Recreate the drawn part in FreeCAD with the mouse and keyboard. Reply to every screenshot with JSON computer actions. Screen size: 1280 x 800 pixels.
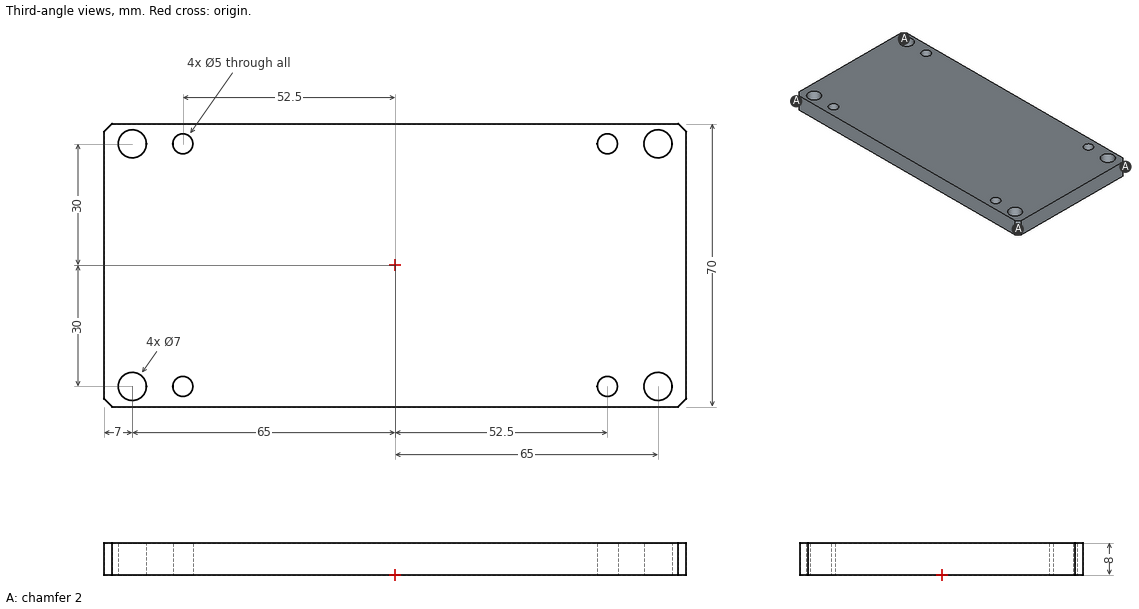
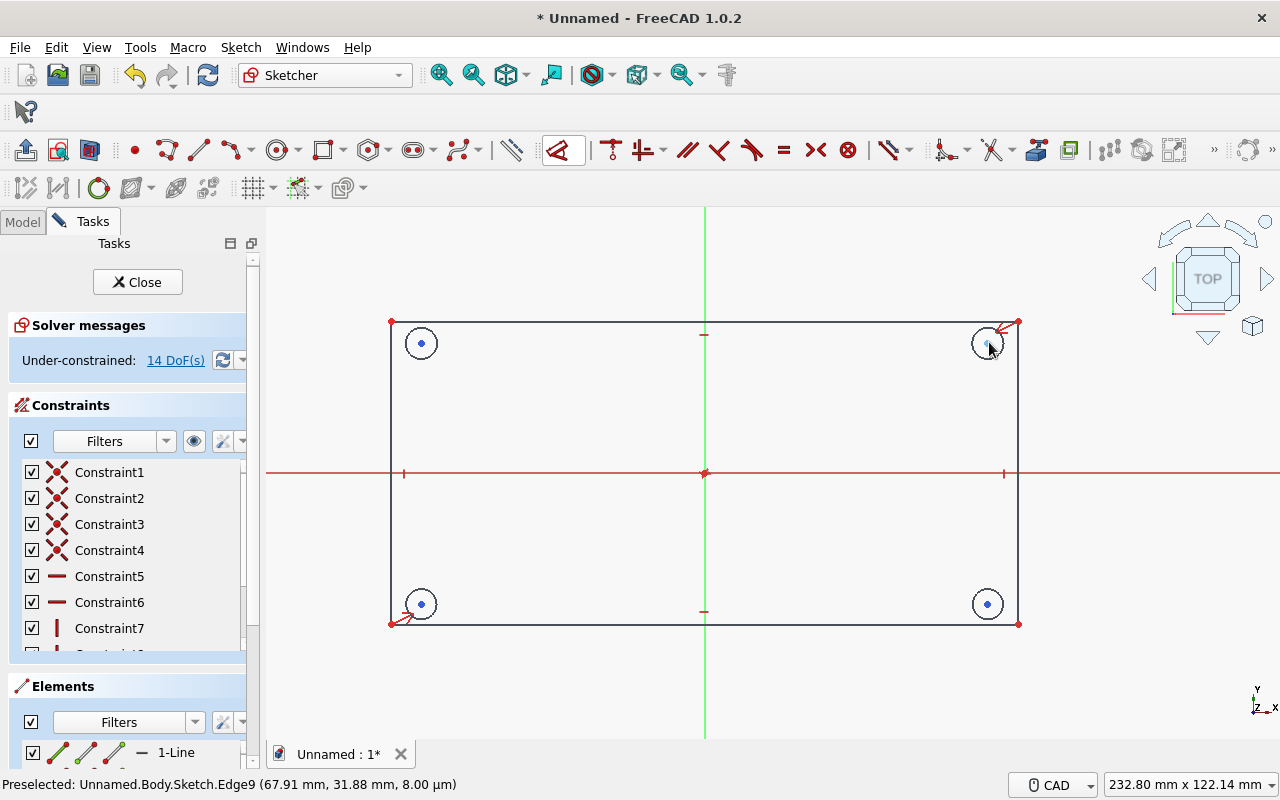
{"action": "left_click", "coordinate": [432, 593]}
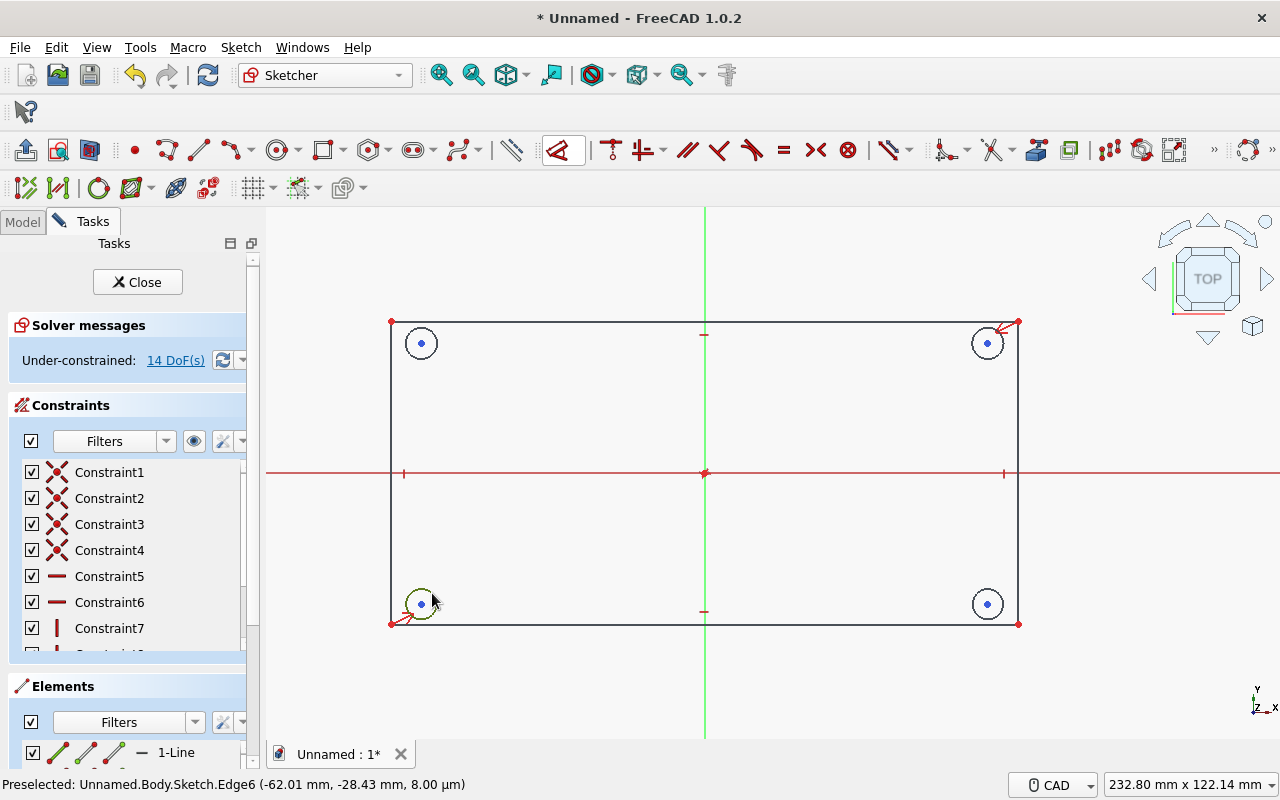
{"action": "left_click", "coordinate": [999, 593]}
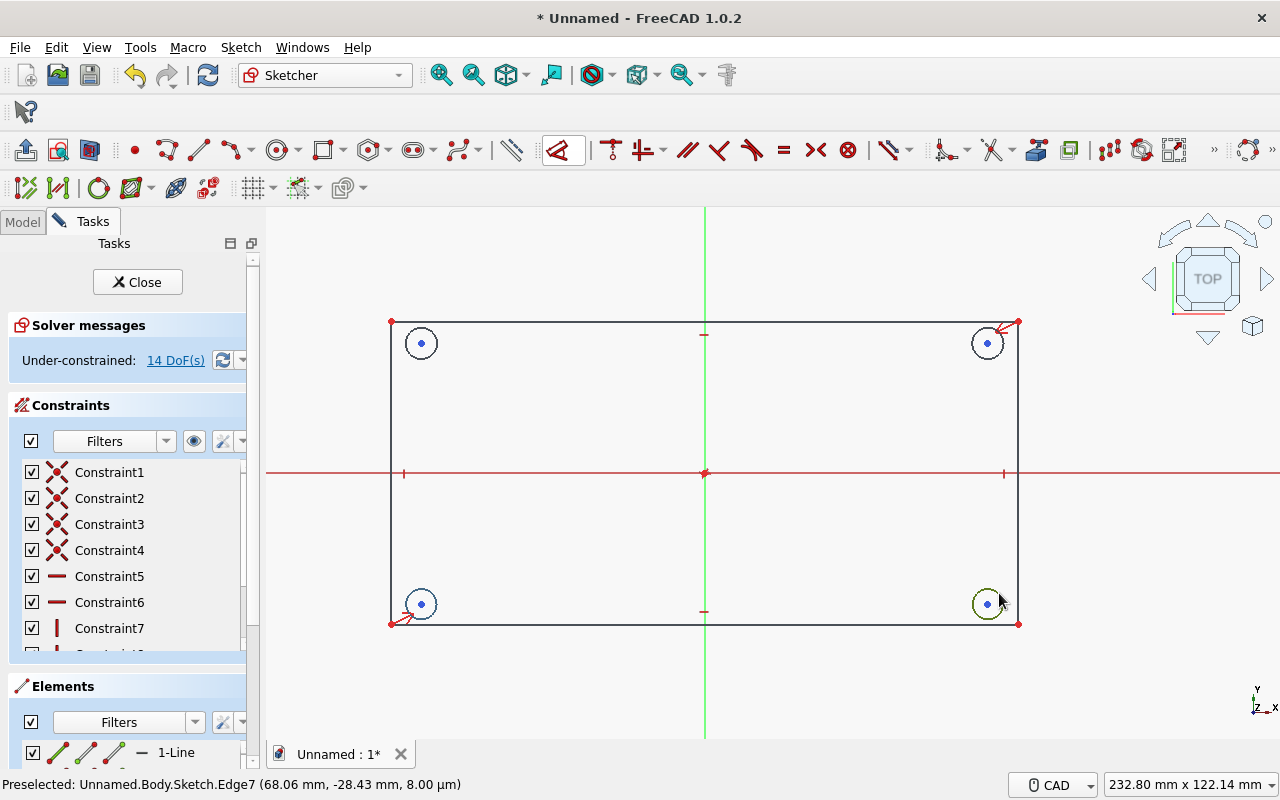
{"action": "scroll", "coordinate": [432, 332], "scroll_direction": "up", "scroll_amount": 2}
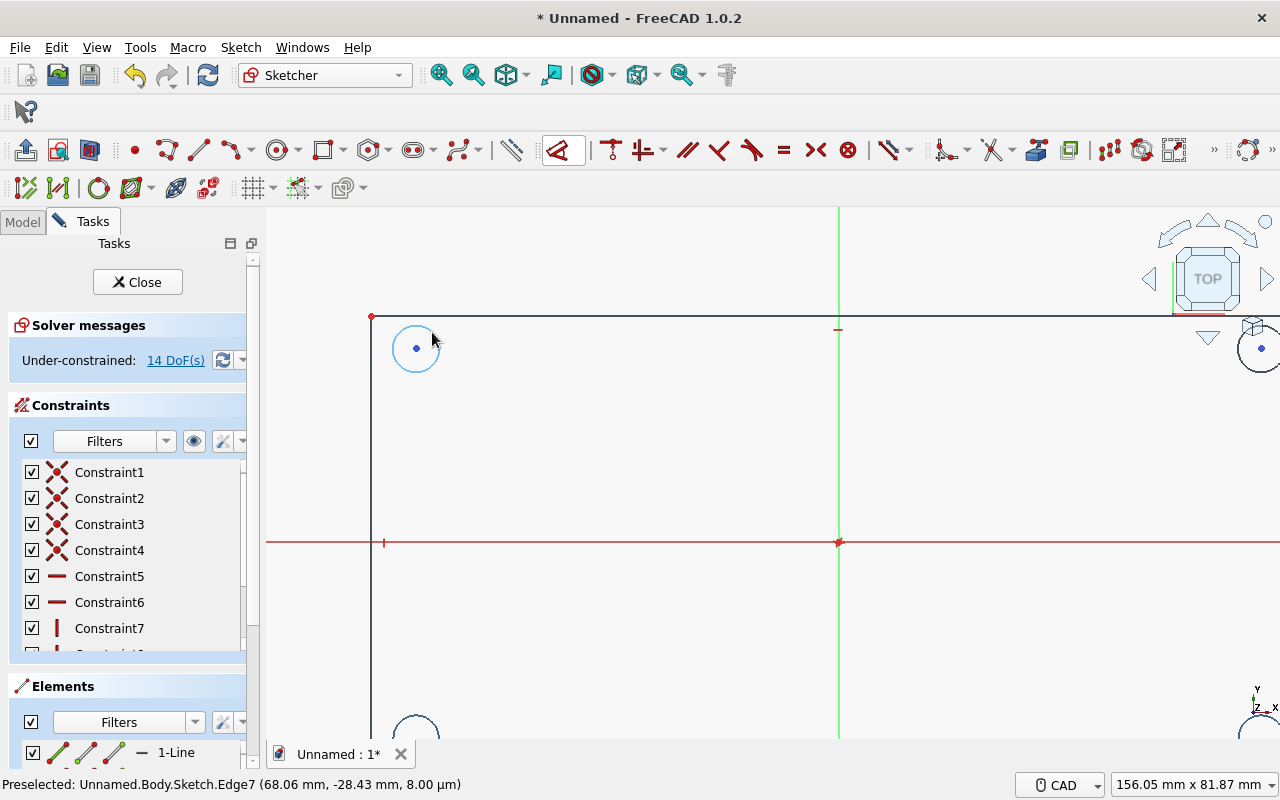
{"action": "left_click", "coordinate": [433, 332]}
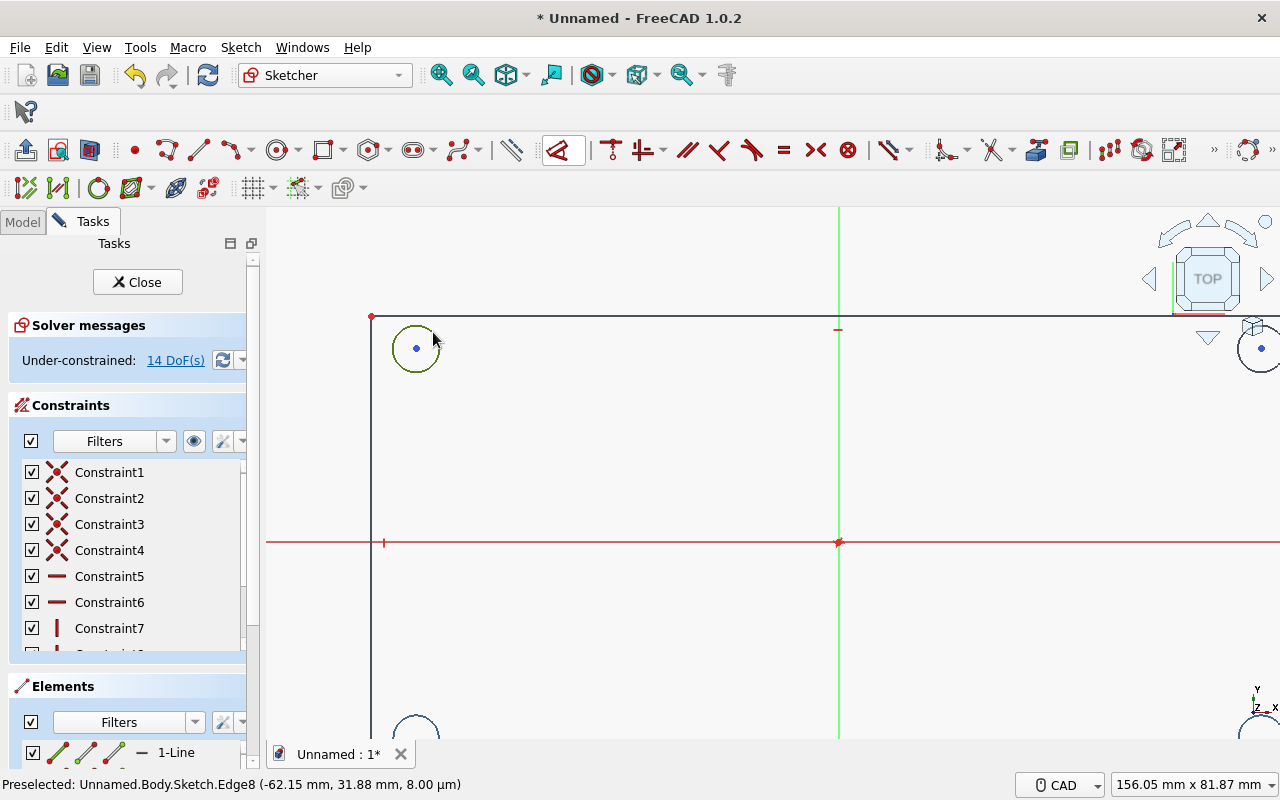
{"action": "scroll", "coordinate": [431, 332], "scroll_direction": "down", "scroll_amount": 2}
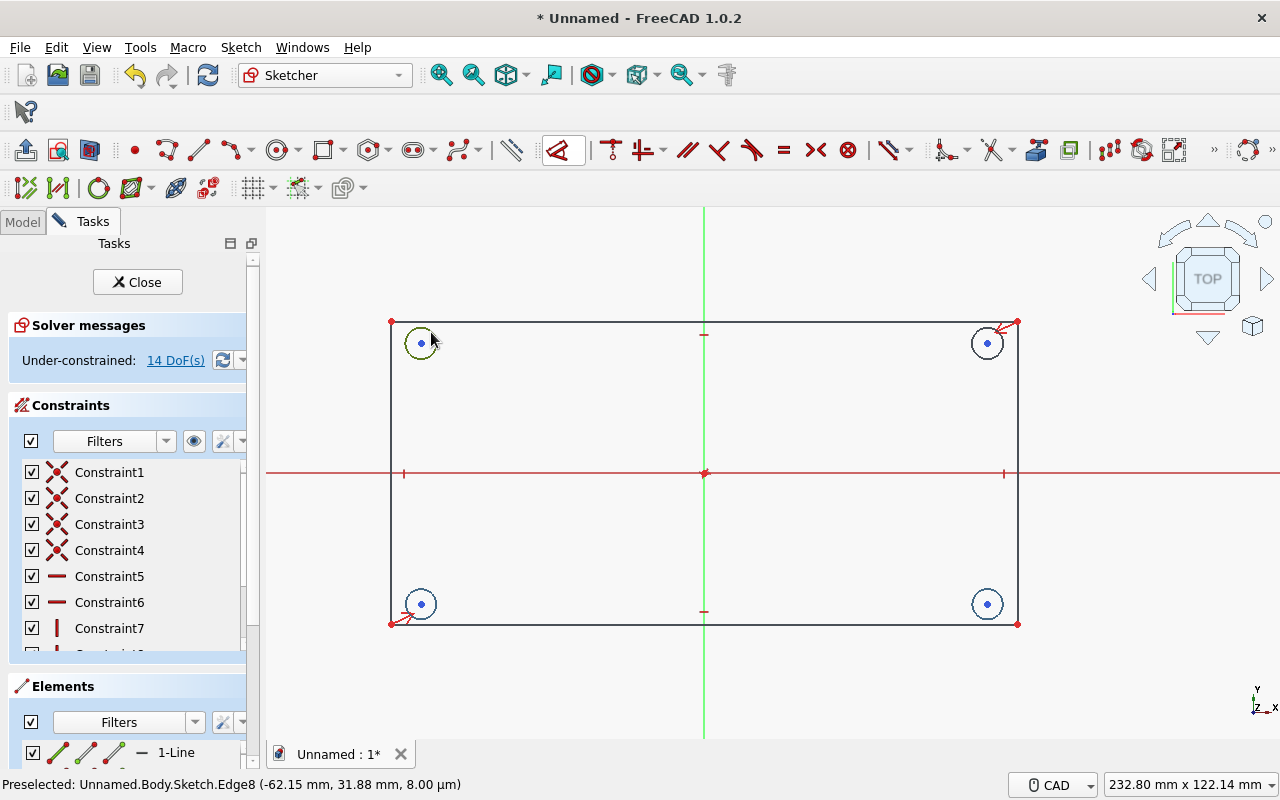
{"action": "scroll", "coordinate": [999, 332], "scroll_direction": "up", "scroll_amount": 2}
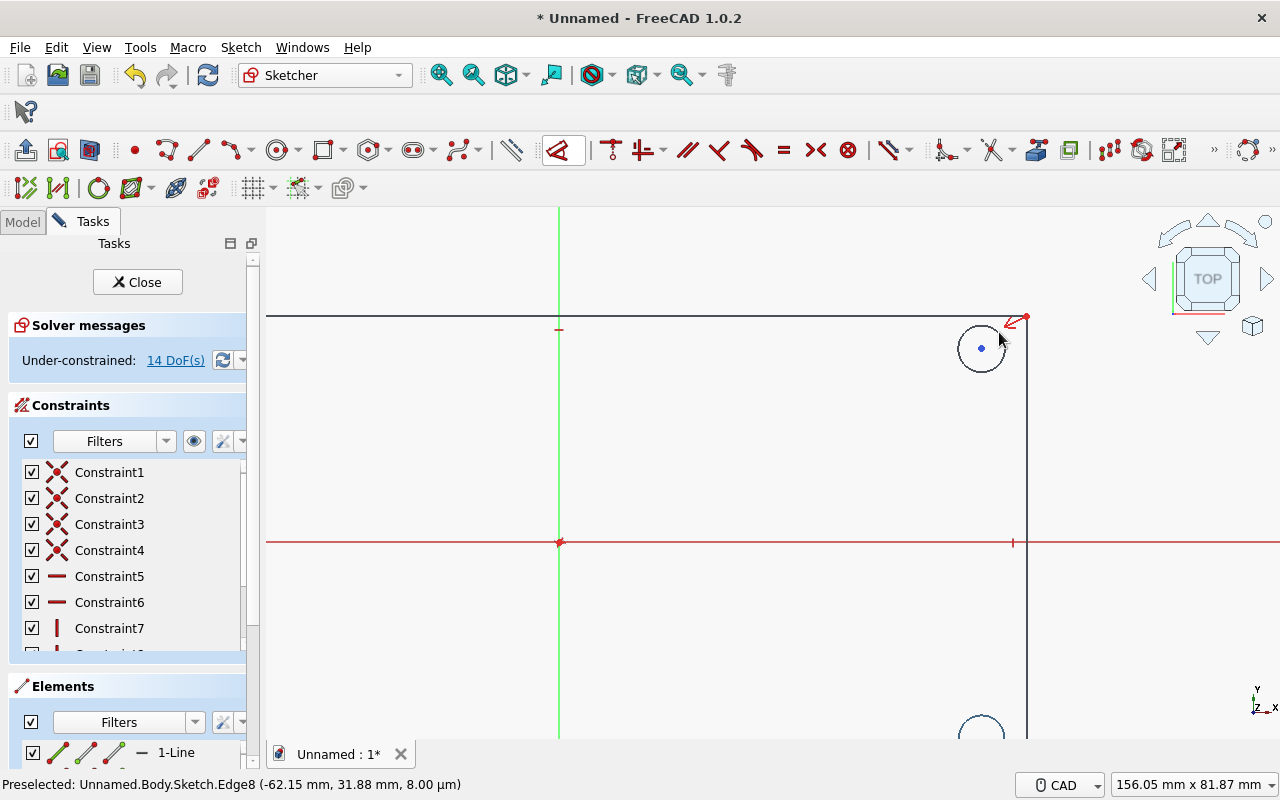
{"action": "left_click", "coordinate": [998, 332]}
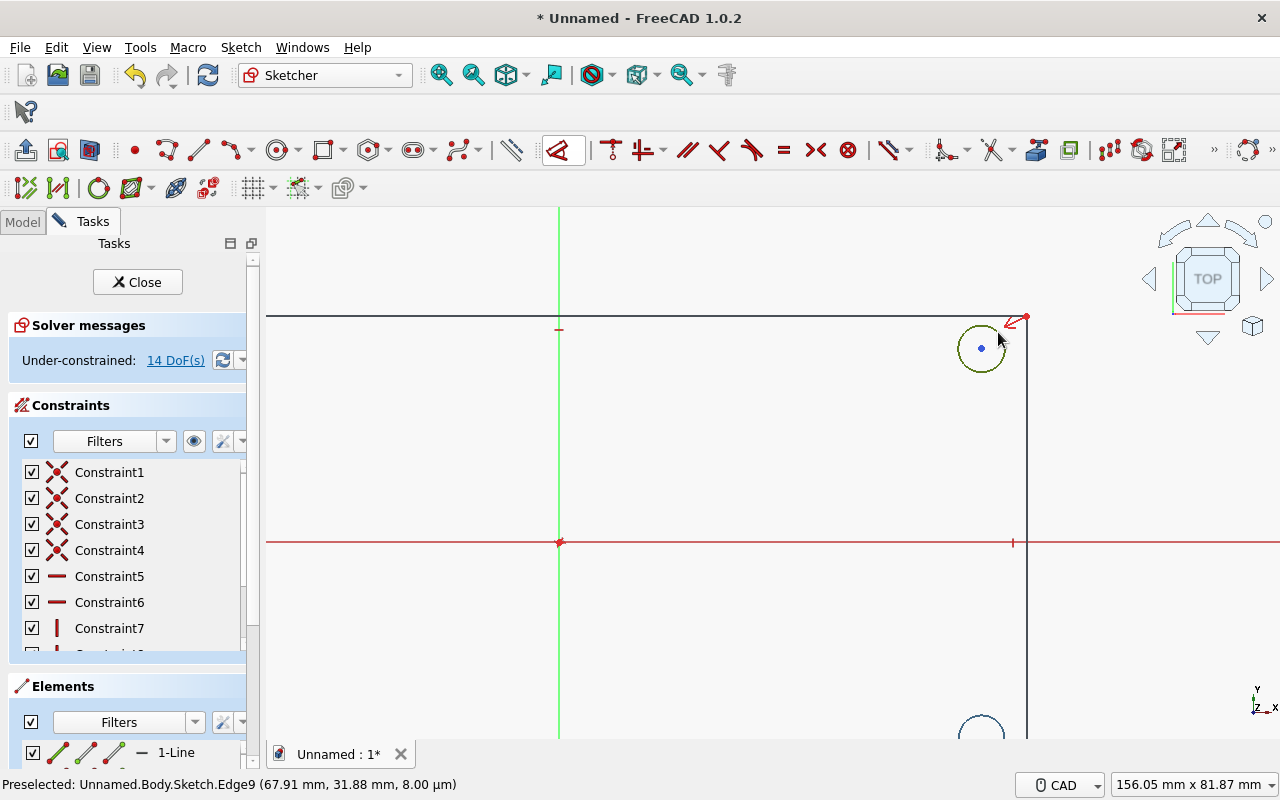
{"action": "left_click", "coordinate": [784, 150]}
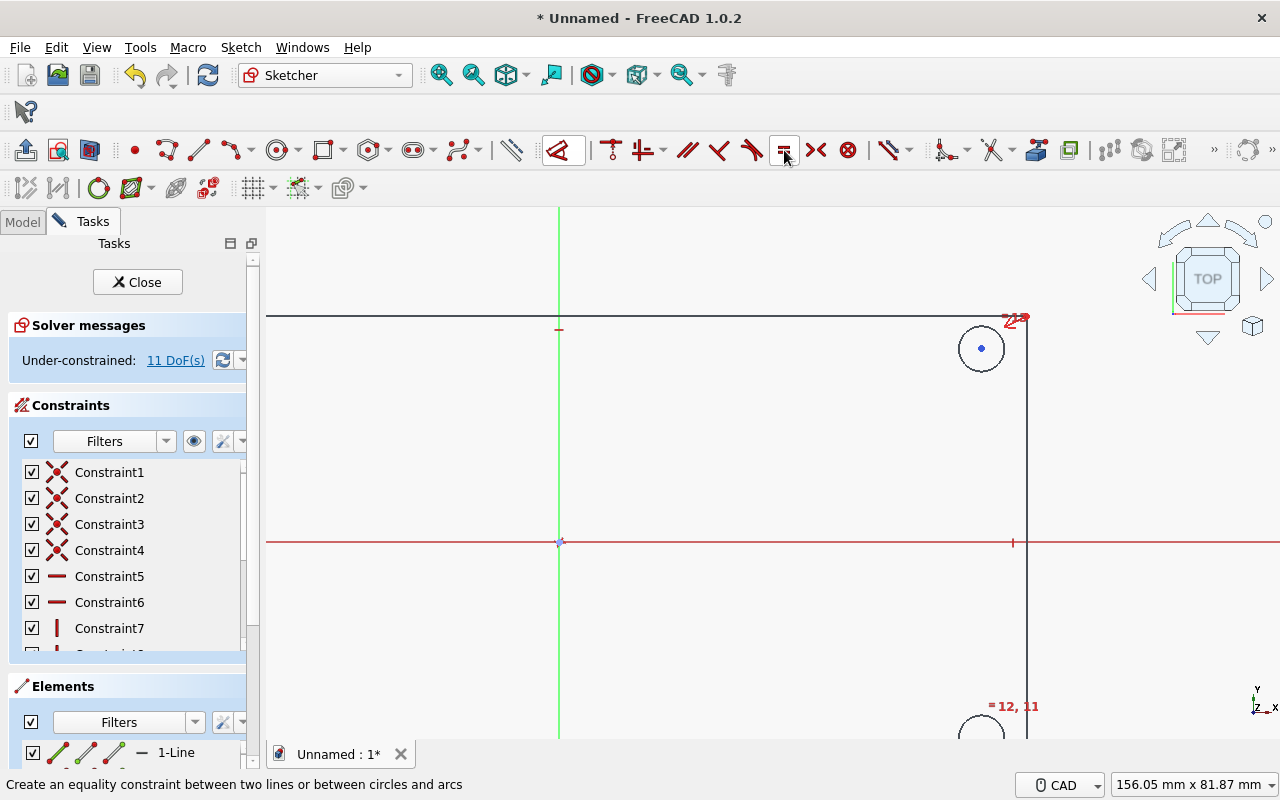
{"action": "scroll", "coordinate": [1000, 332], "scroll_direction": "down", "scroll_amount": 2}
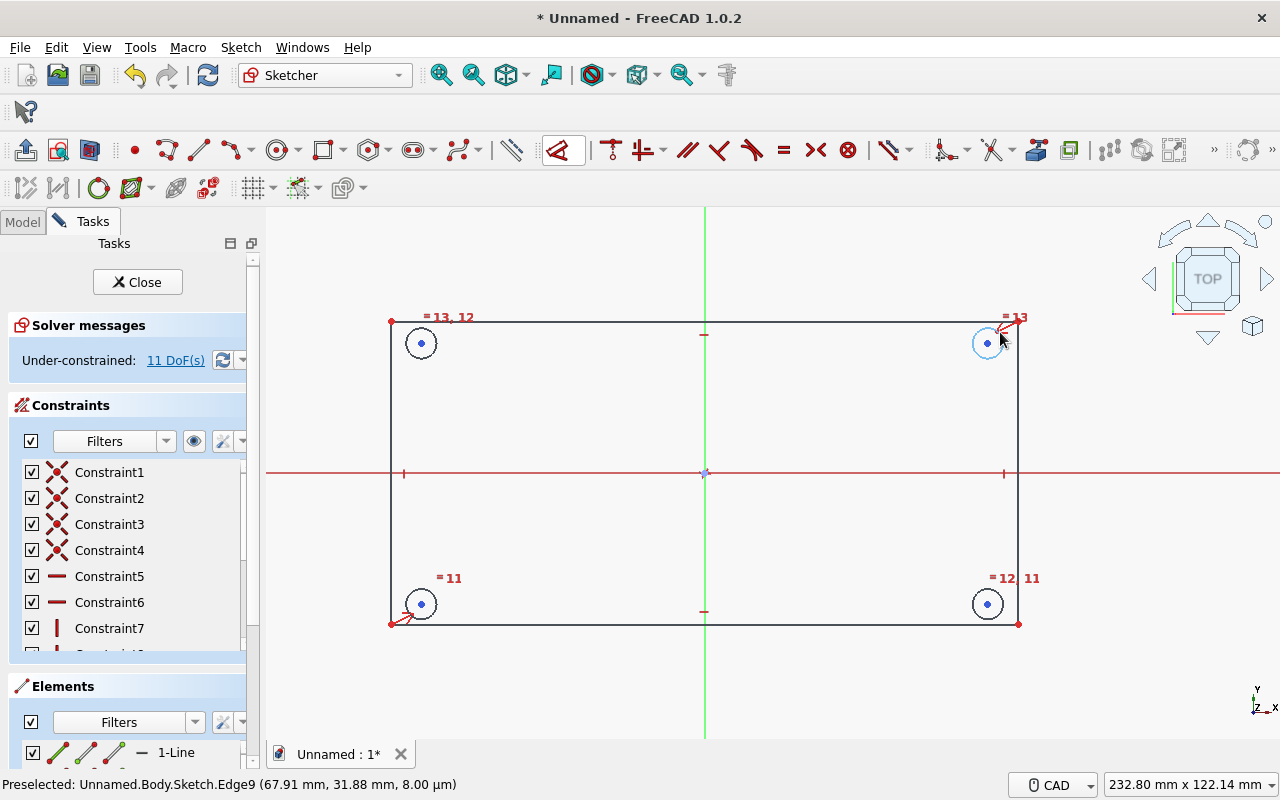
{"action": "scroll", "coordinate": [432, 593], "scroll_direction": "up", "scroll_amount": 2}